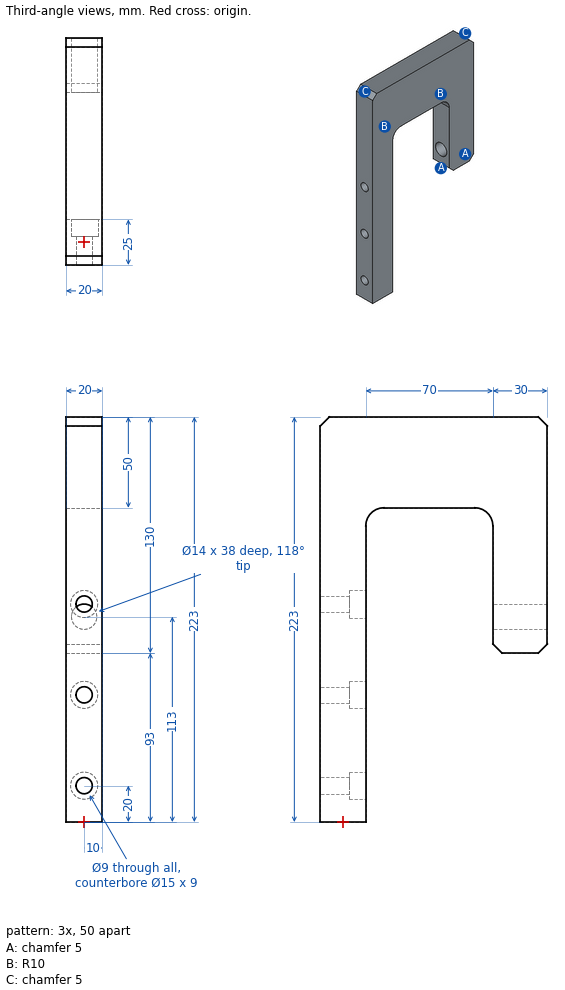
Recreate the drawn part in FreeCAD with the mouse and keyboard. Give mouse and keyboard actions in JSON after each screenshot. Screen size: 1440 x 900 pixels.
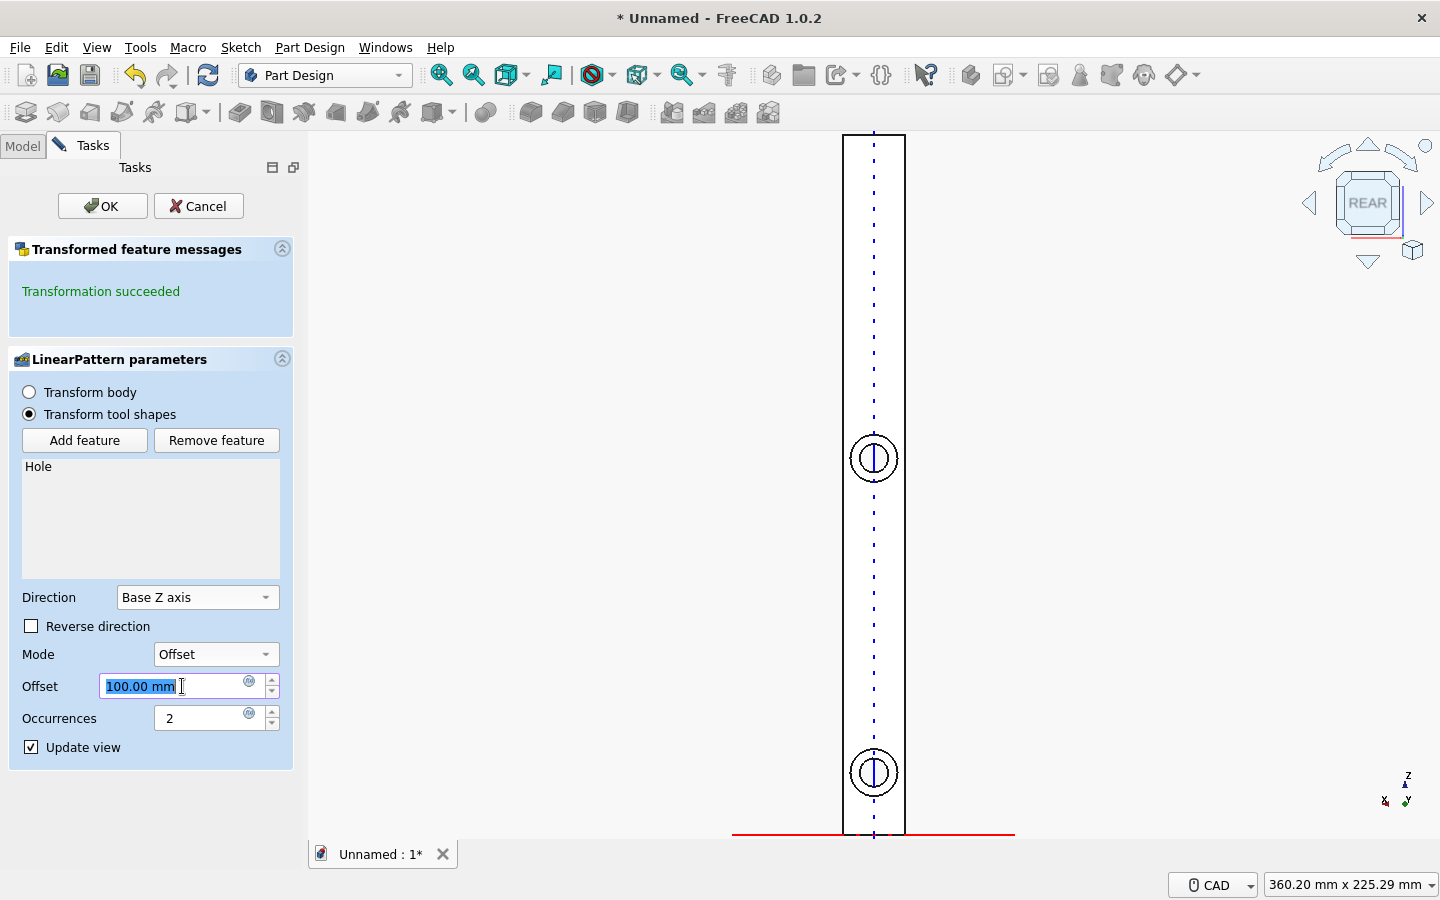
{"action": "type", "text": "50"}
{"action": "key", "text": "Tab"}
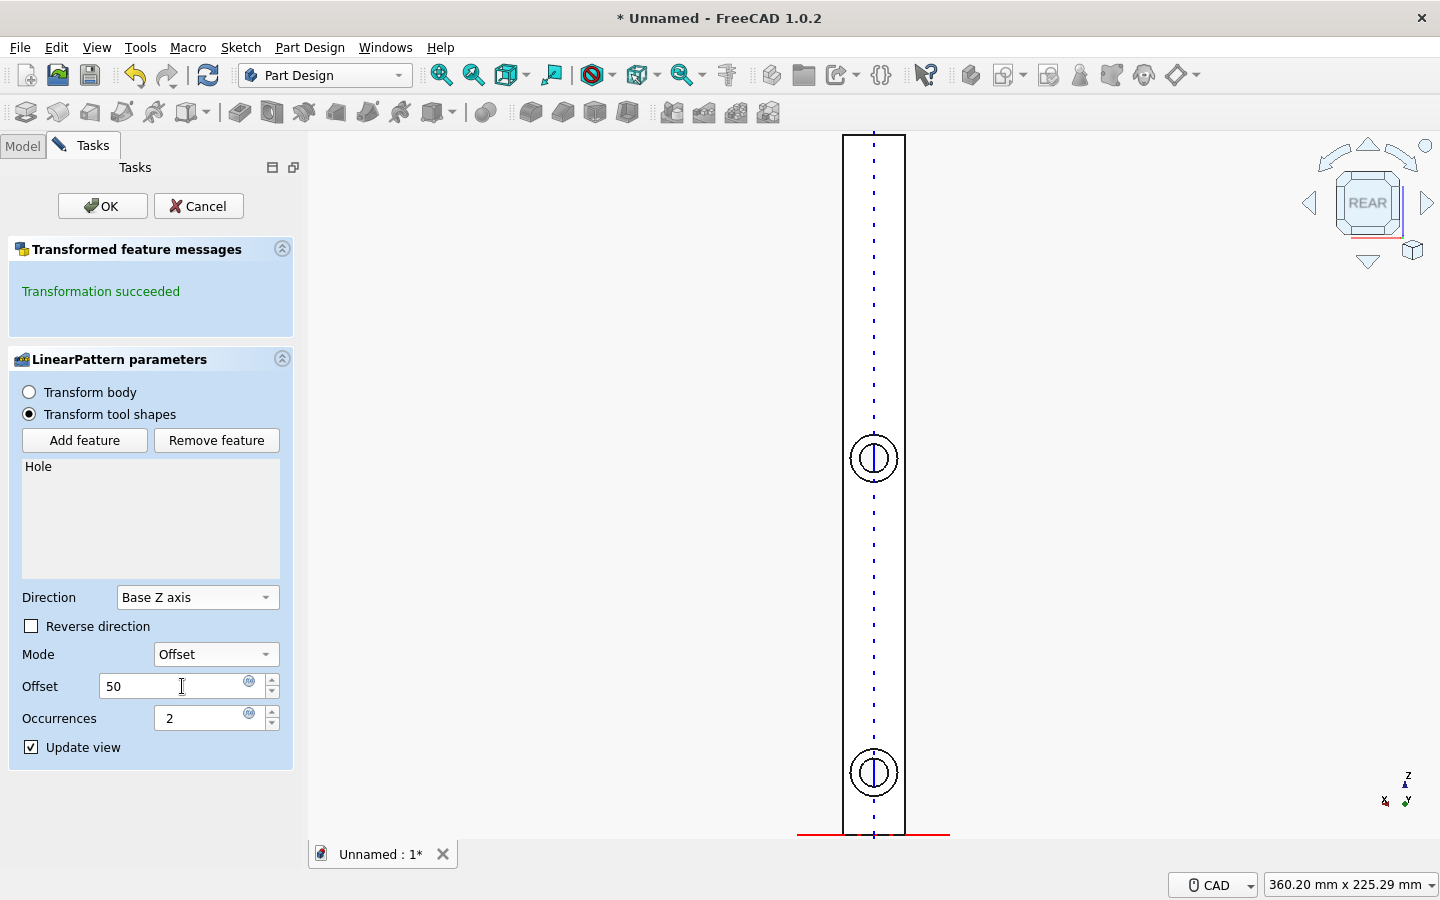
{"action": "triple_click", "coordinate": [209, 718]}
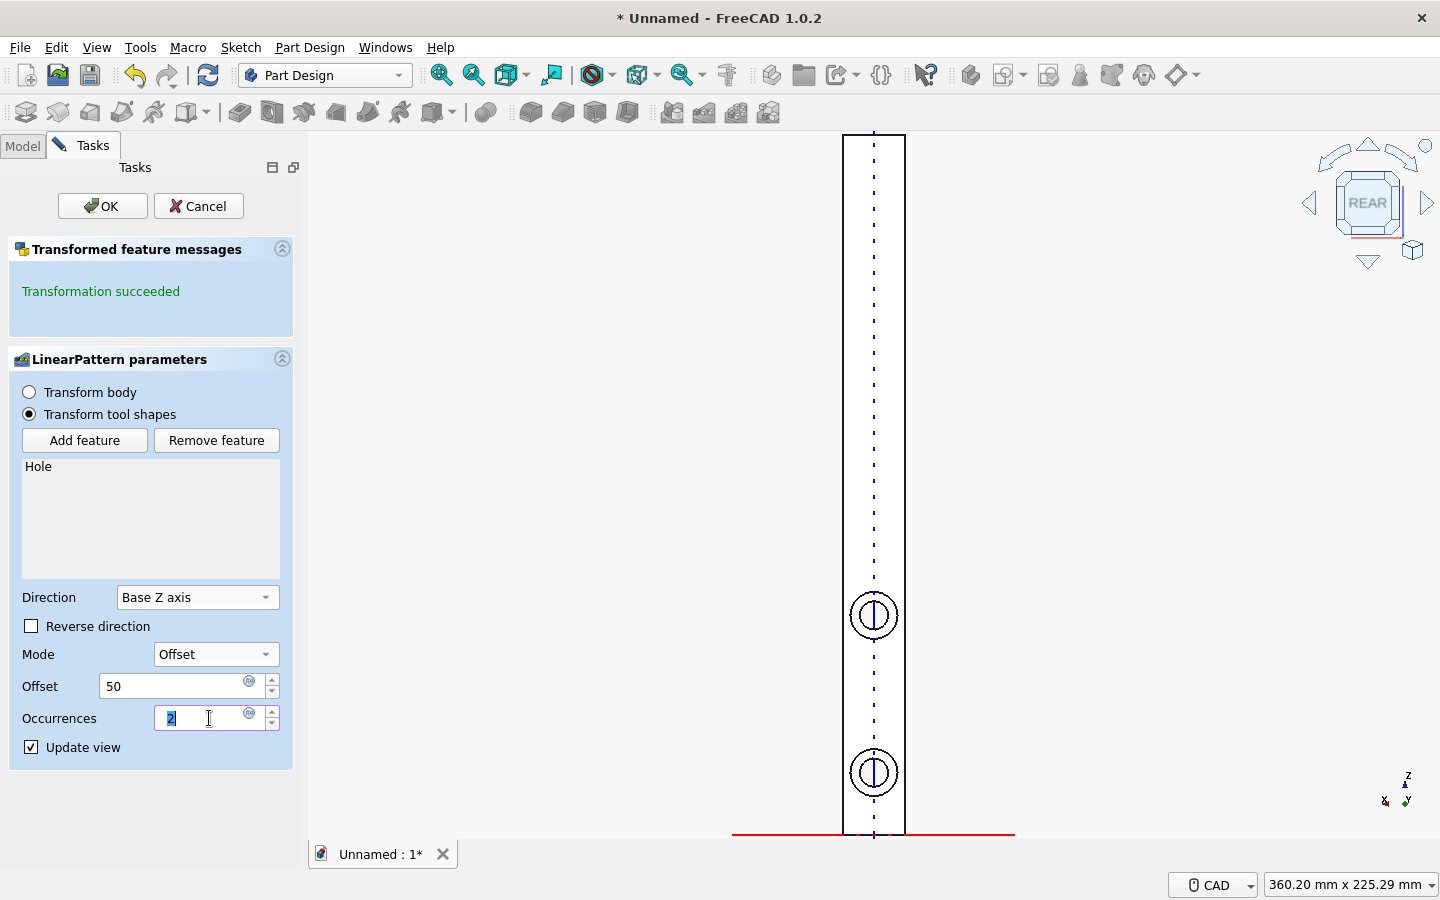
{"action": "type", "text": "3"}
{"action": "key", "text": "Tab"}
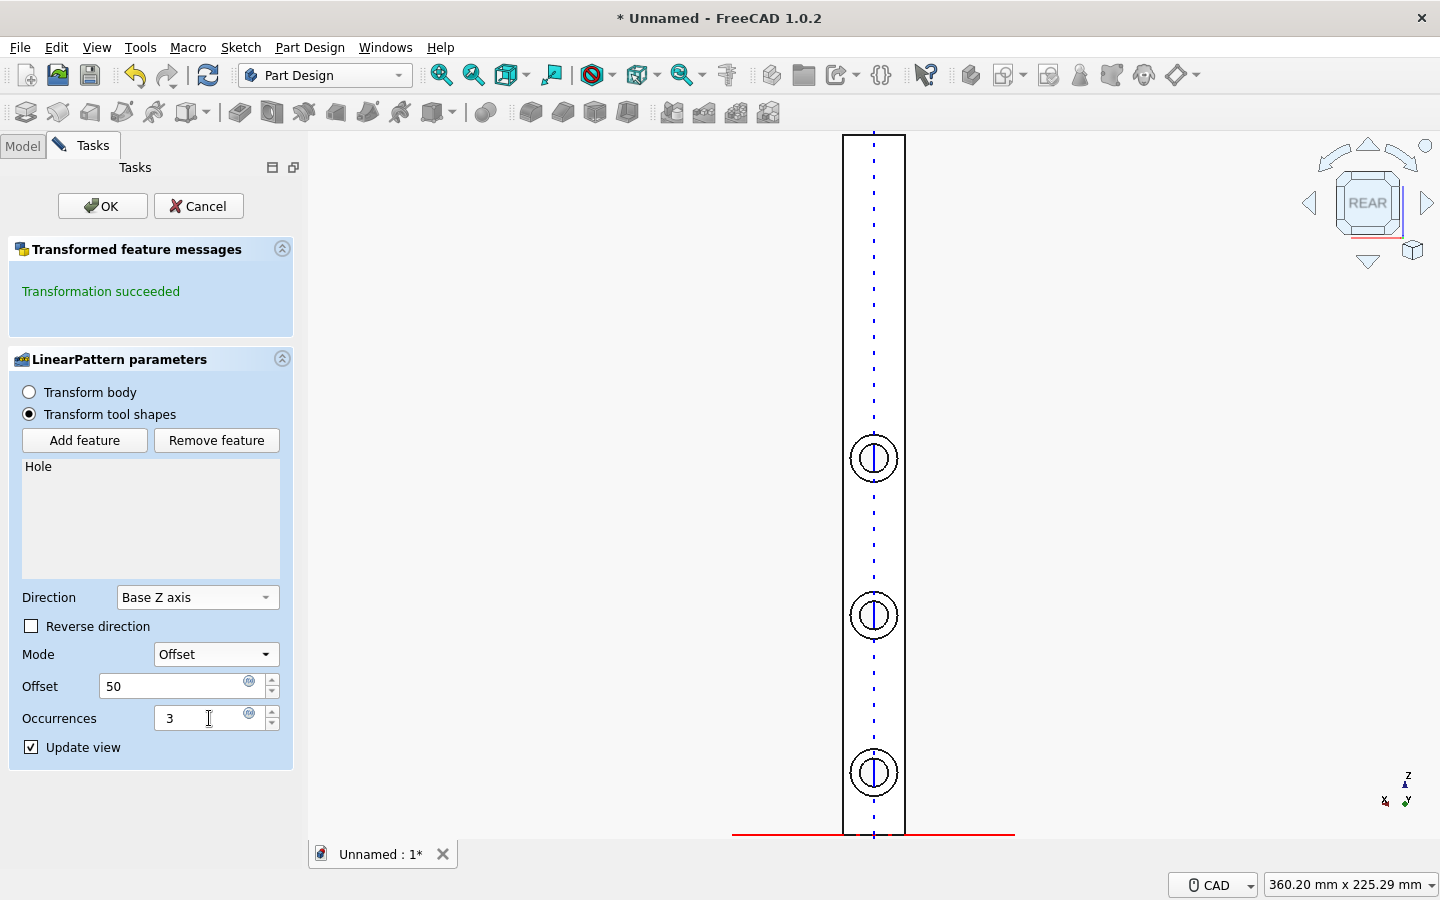
{"action": "left_click", "coordinate": [103, 206]}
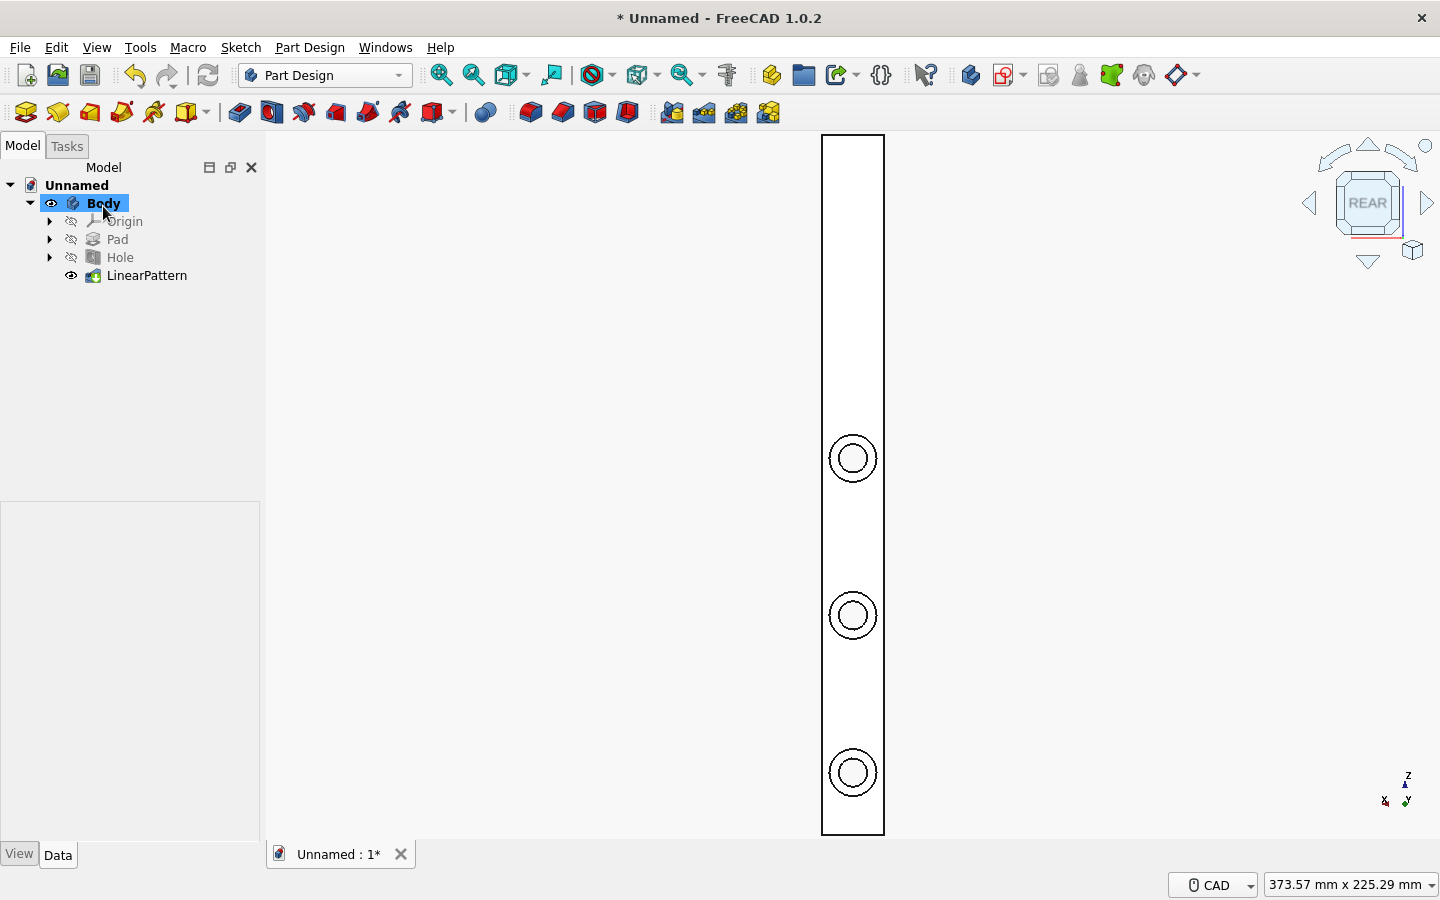
{"action": "left_click", "coordinate": [853, 184]}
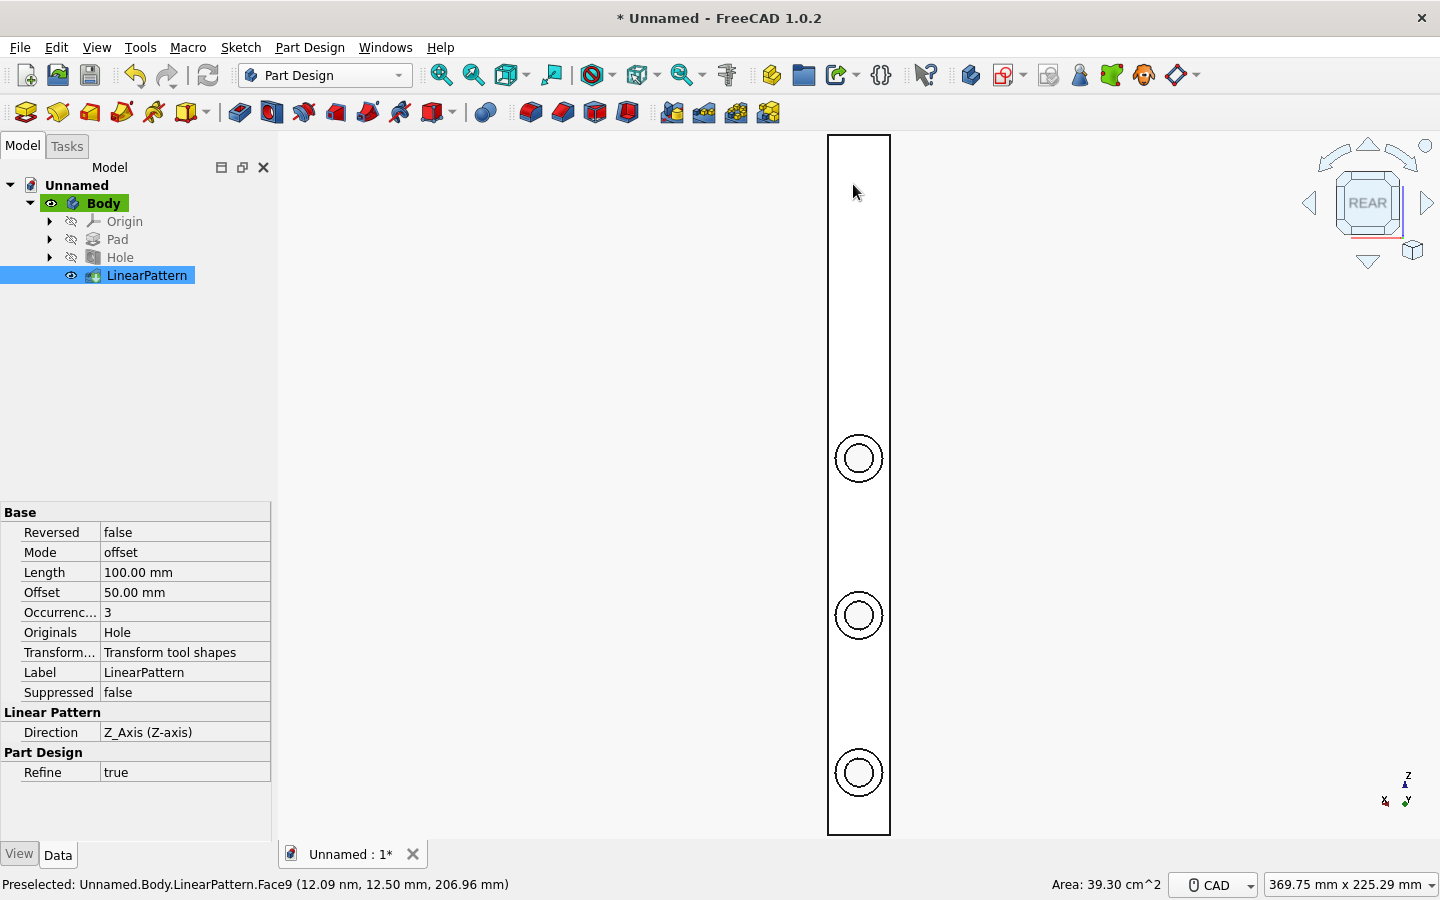
{"action": "left_click", "coordinate": [1004, 76]}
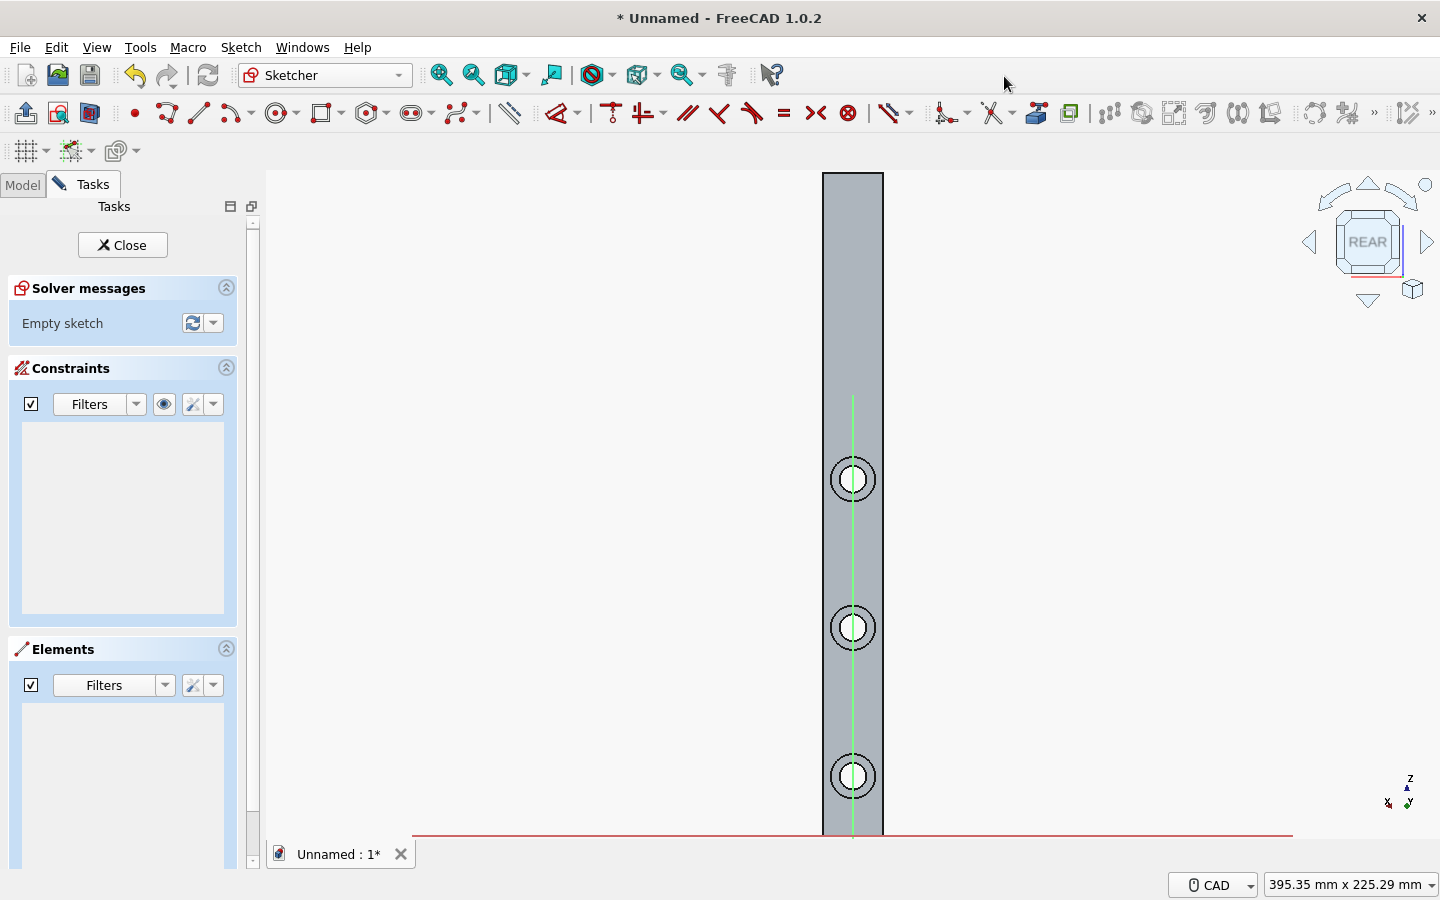
{"action": "scroll", "coordinate": [784, 504], "scroll_direction": "down", "scroll_amount": 5}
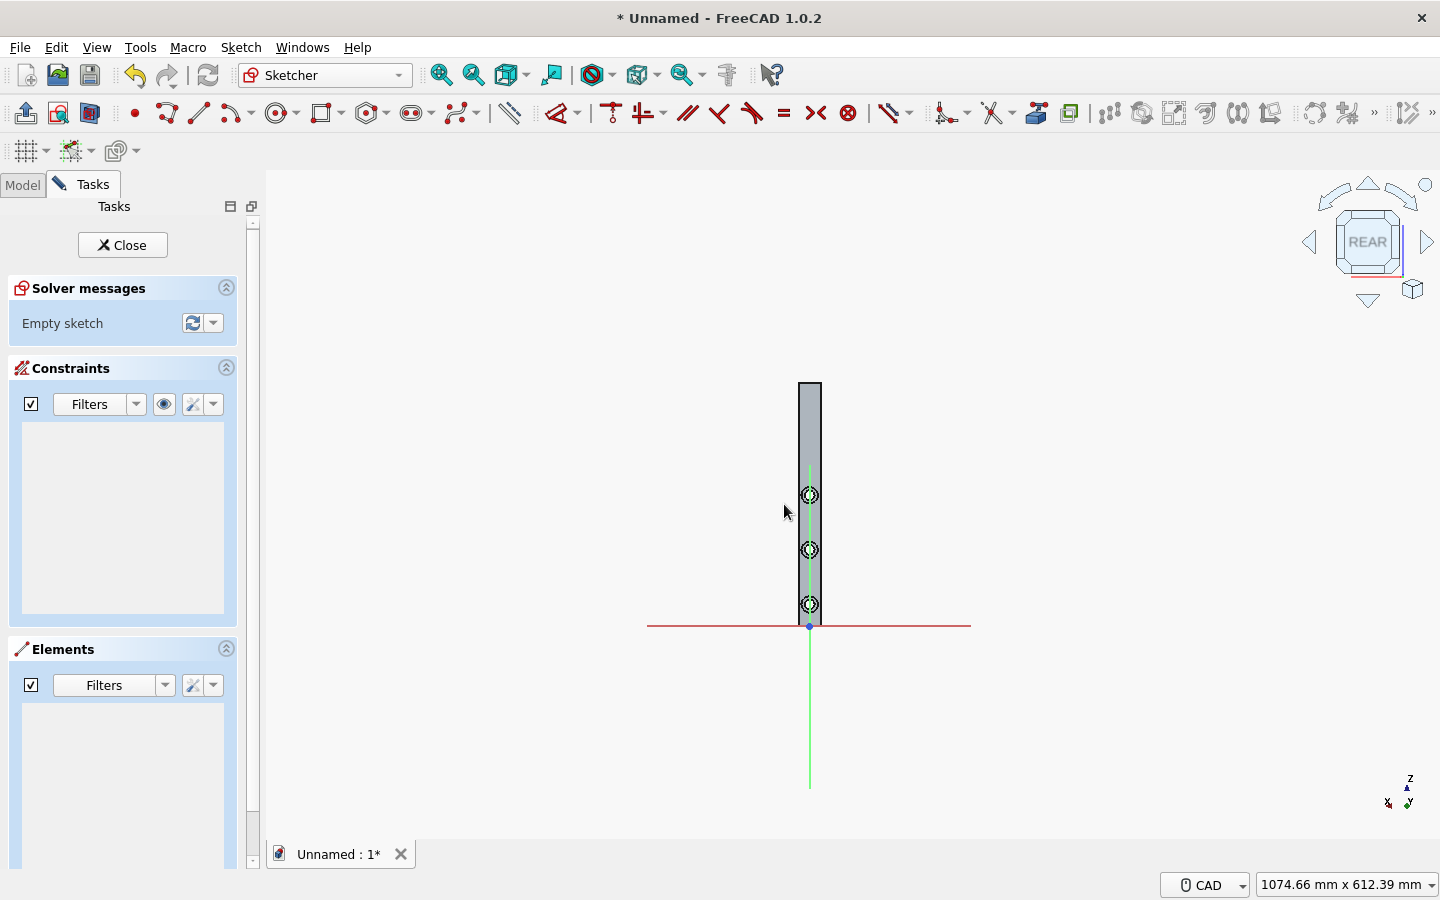
{"action": "scroll", "coordinate": [814, 395], "scroll_direction": "up", "scroll_amount": 10}